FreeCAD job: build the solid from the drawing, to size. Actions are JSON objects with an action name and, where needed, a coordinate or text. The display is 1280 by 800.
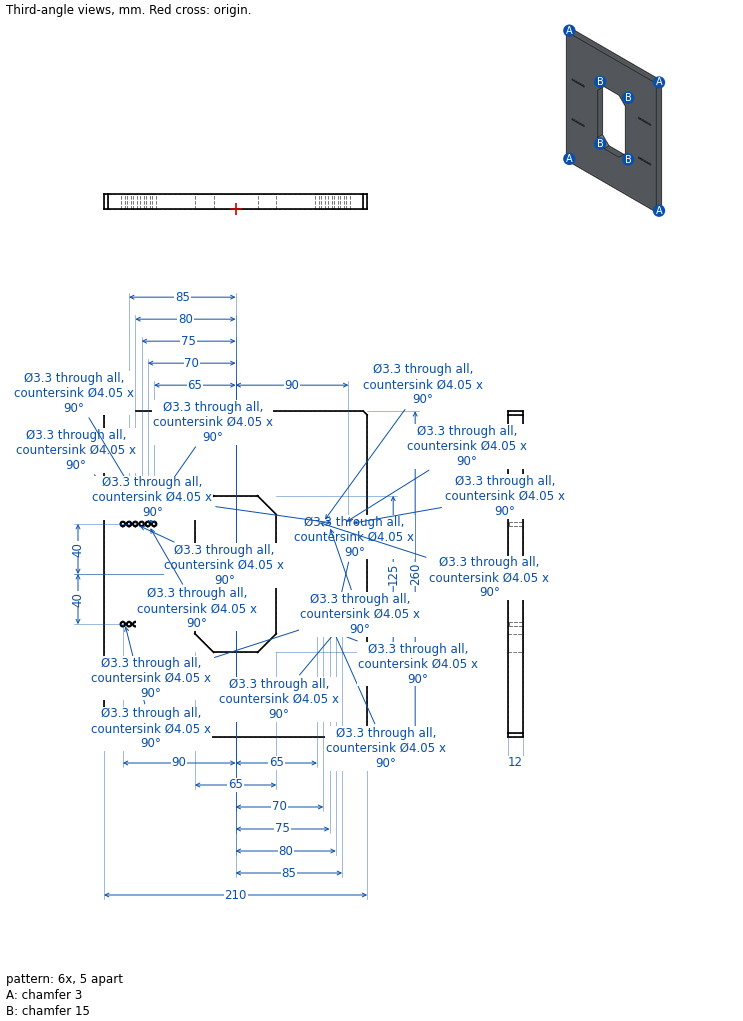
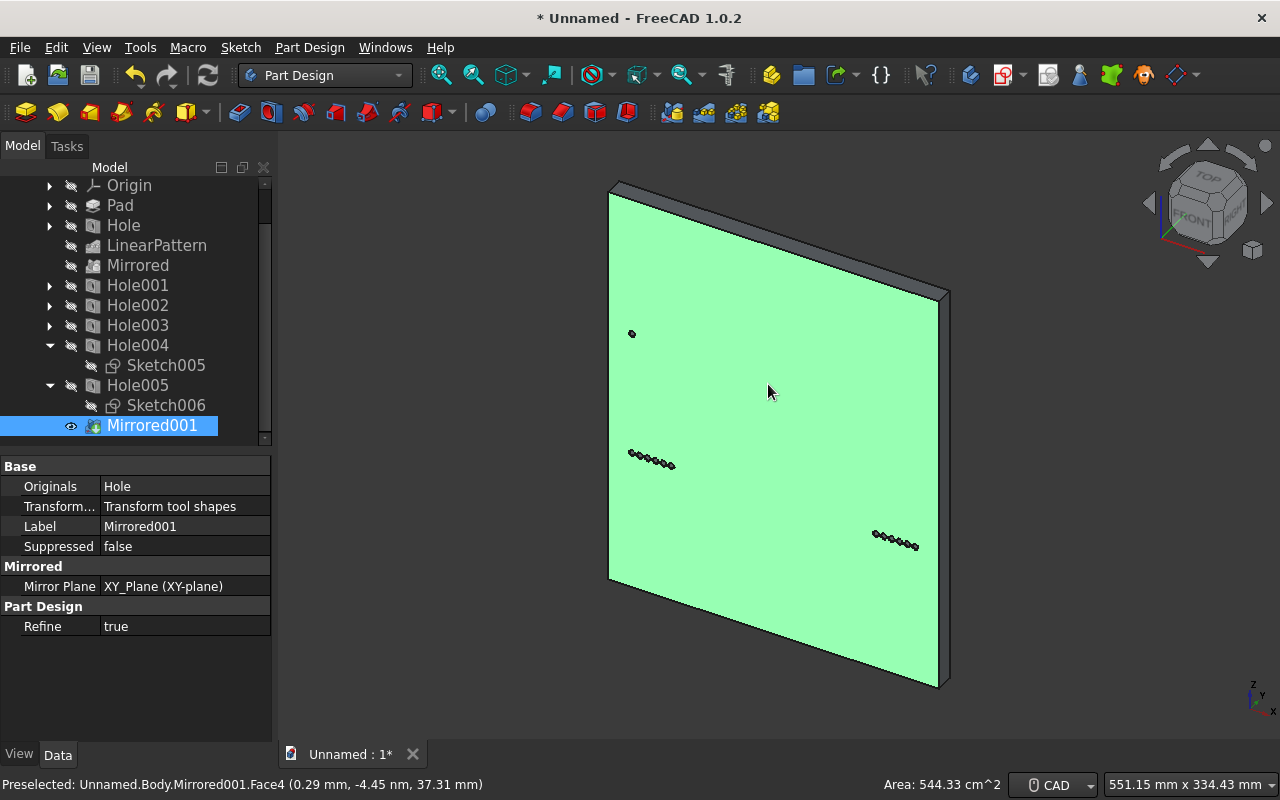
{"action": "left_click", "coordinate": [1004, 76]}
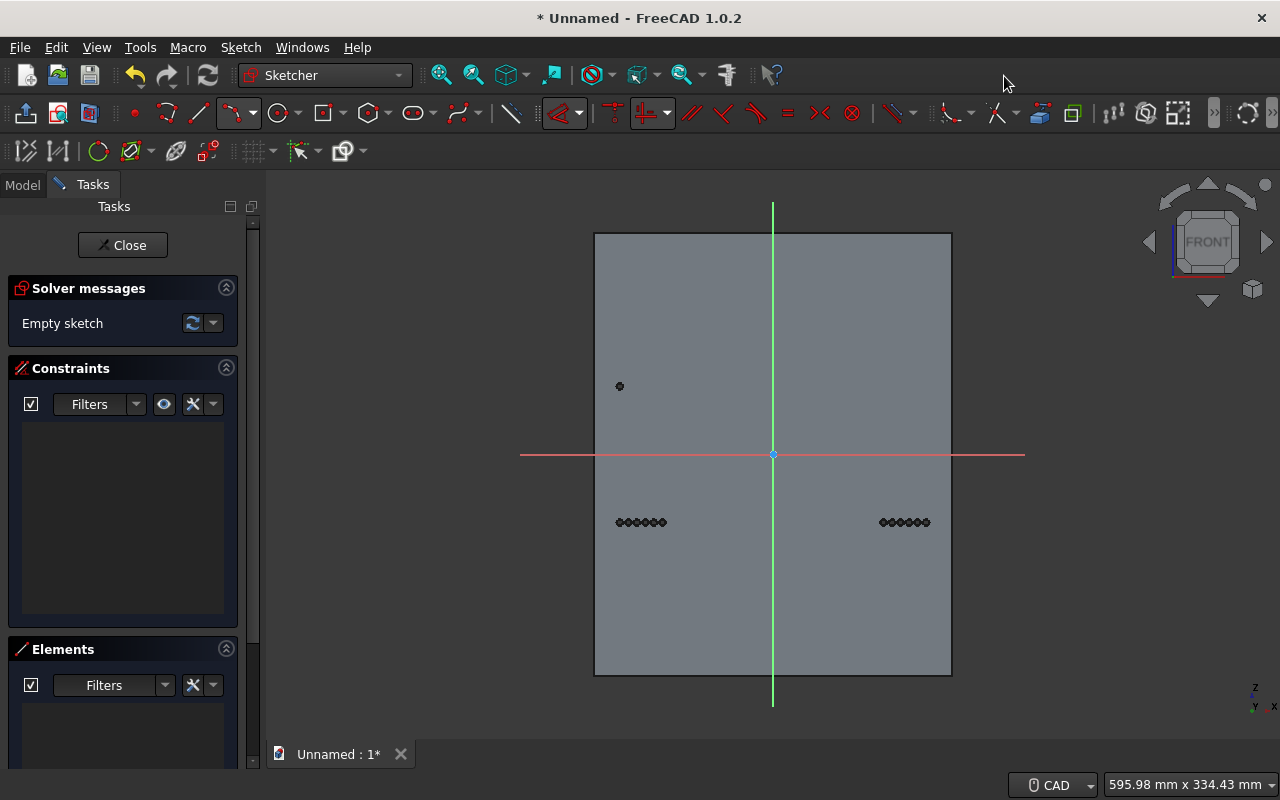
{"action": "scroll", "coordinate": [624, 383], "scroll_direction": "up", "scroll_amount": 15}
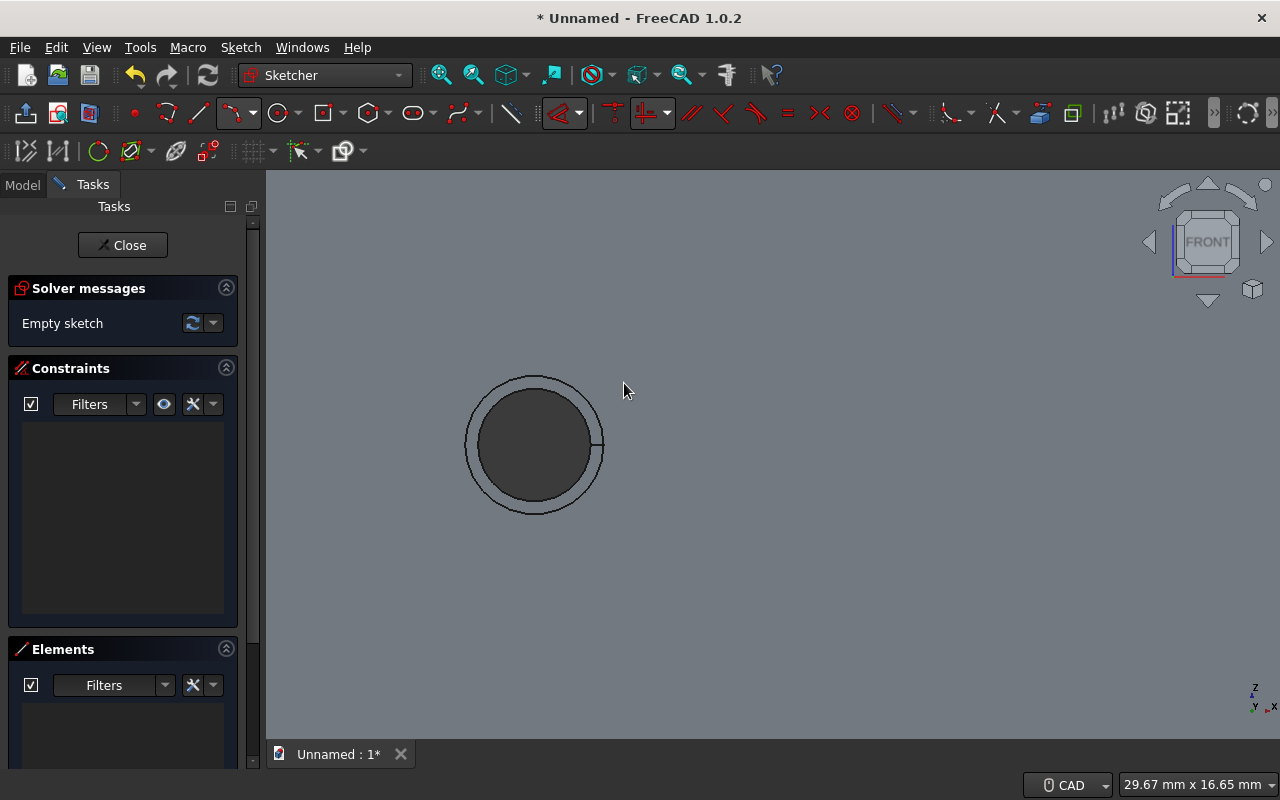
{"action": "scroll", "coordinate": [706, 441], "scroll_direction": "up", "scroll_amount": 6}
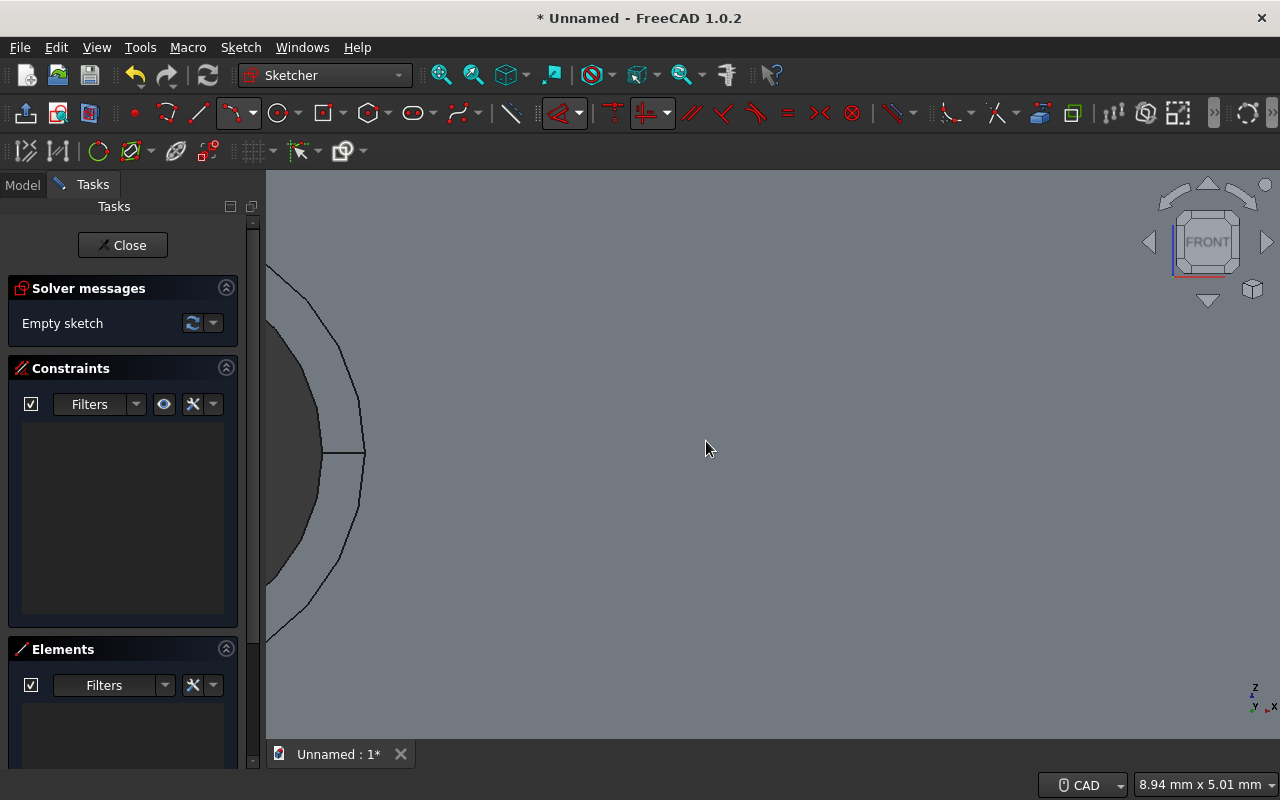
{"action": "left_click", "coordinate": [278, 114]}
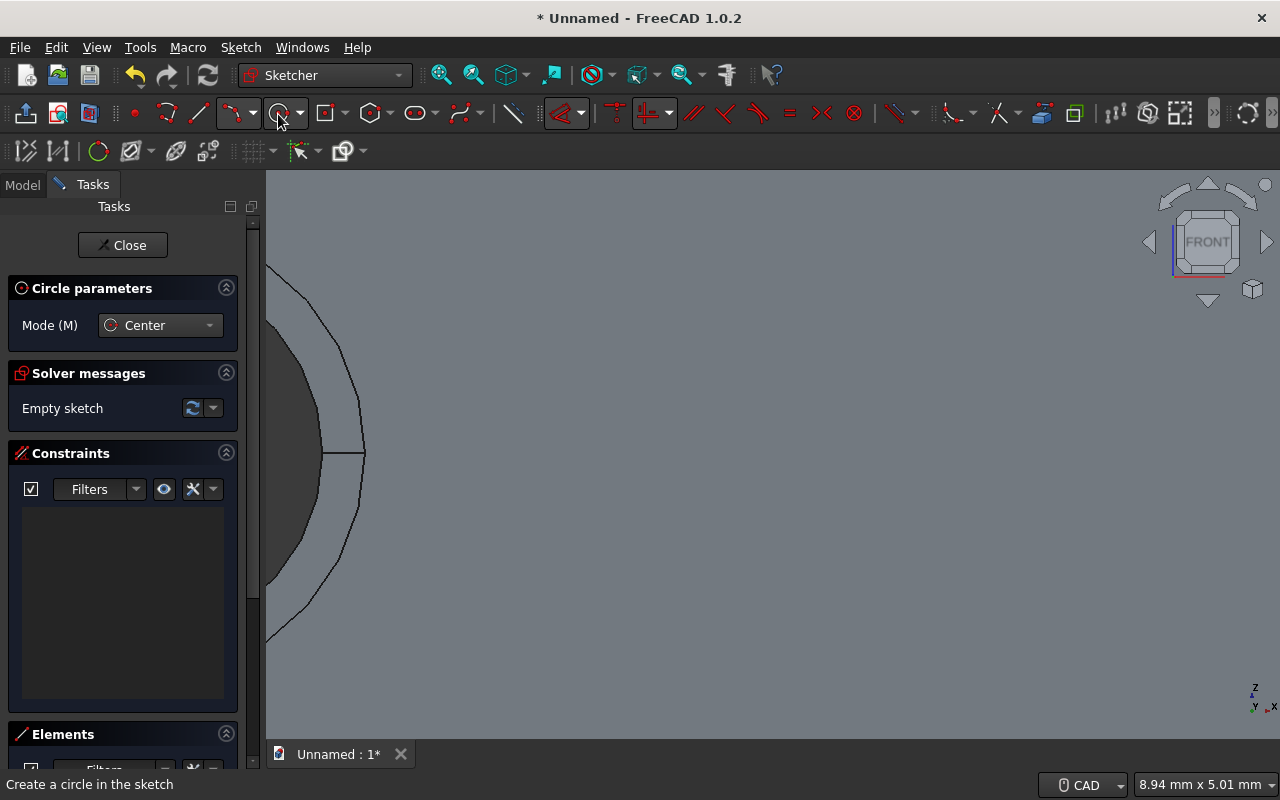
{"action": "left_click", "coordinate": [703, 453]}
{"action": "mouse_move", "coordinate": [835, 321]}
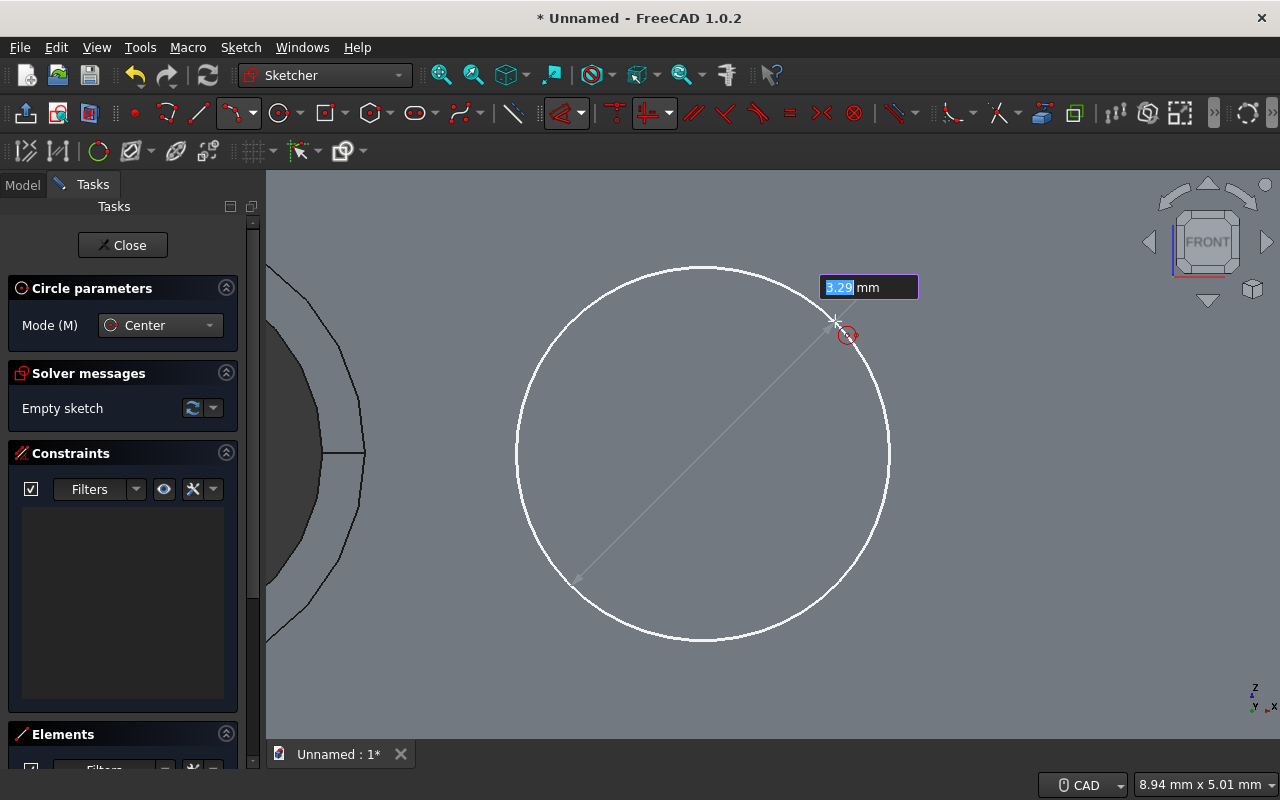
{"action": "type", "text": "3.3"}
{"action": "key", "text": "Return"}
{"action": "key", "text": "Escape"}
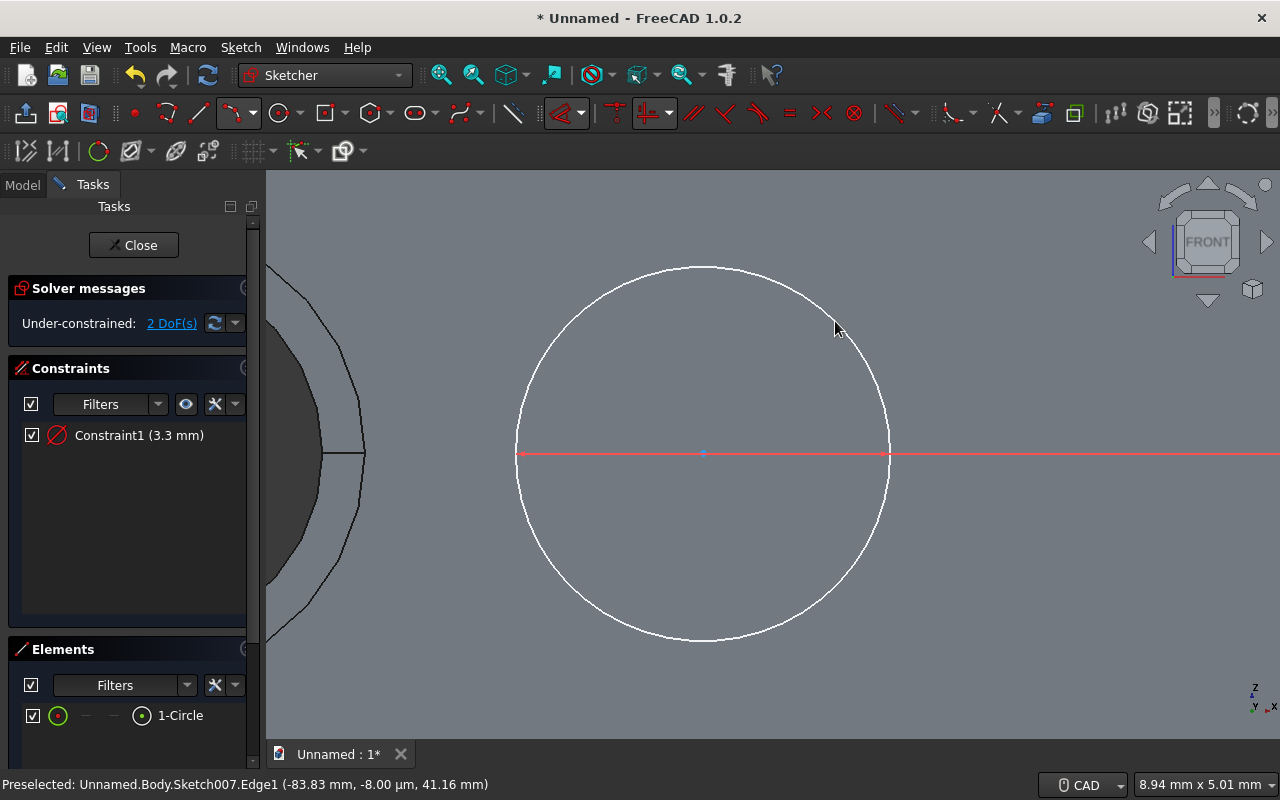
{"action": "left_click", "coordinate": [703, 454]}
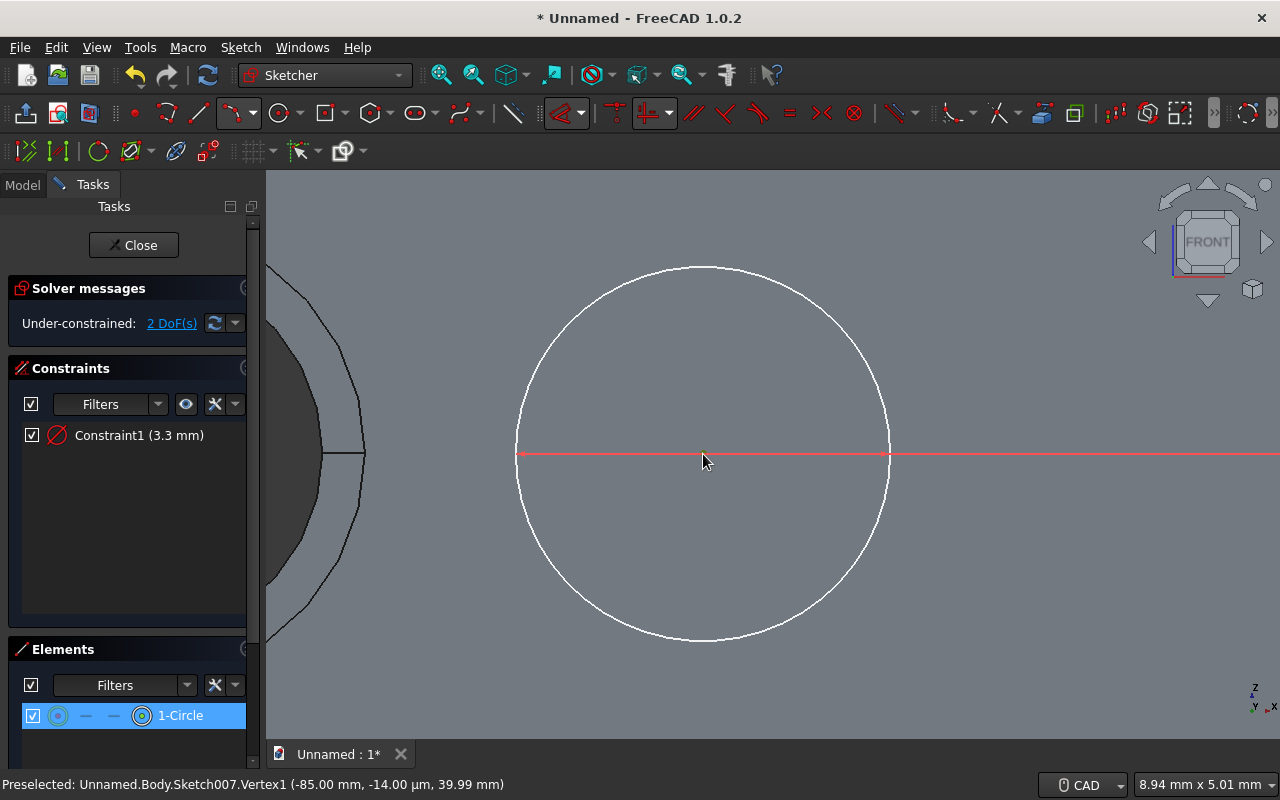
{"action": "left_click", "coordinate": [584, 114]}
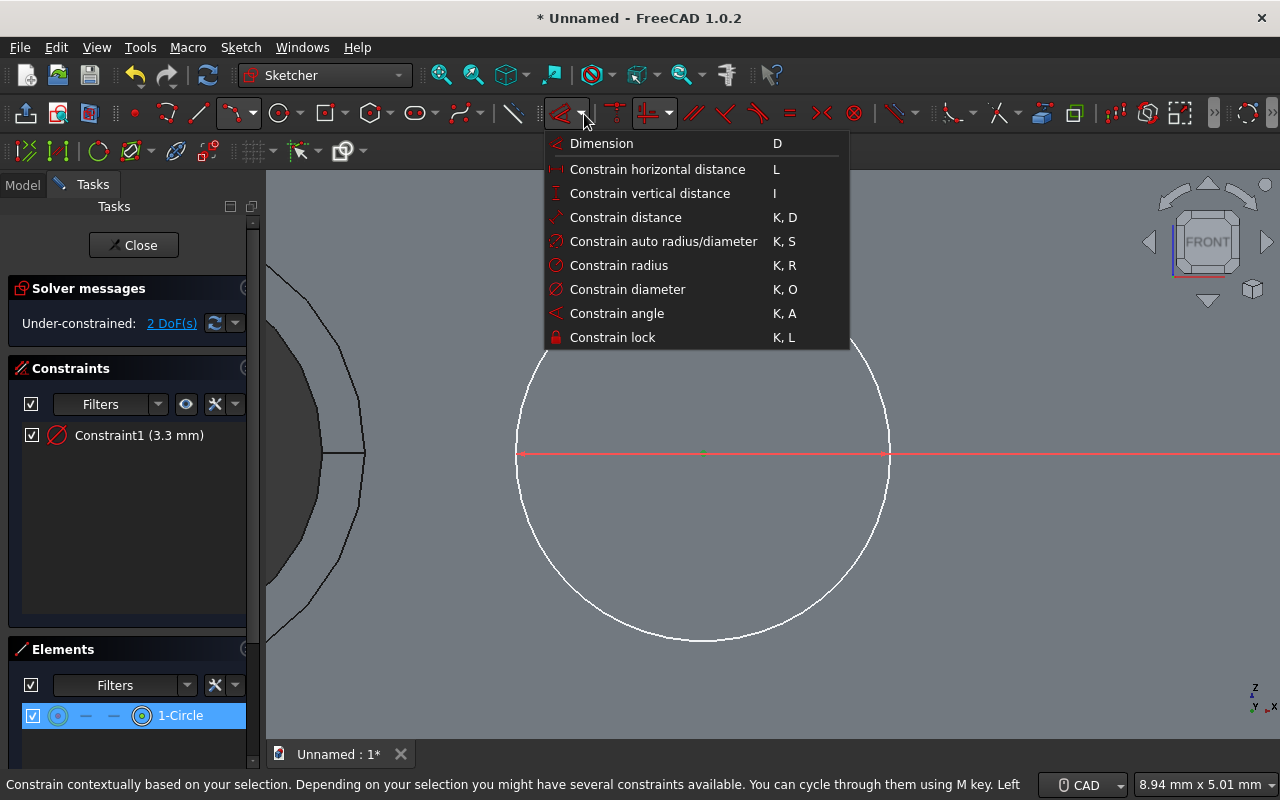
{"action": "left_click", "coordinate": [697, 169]}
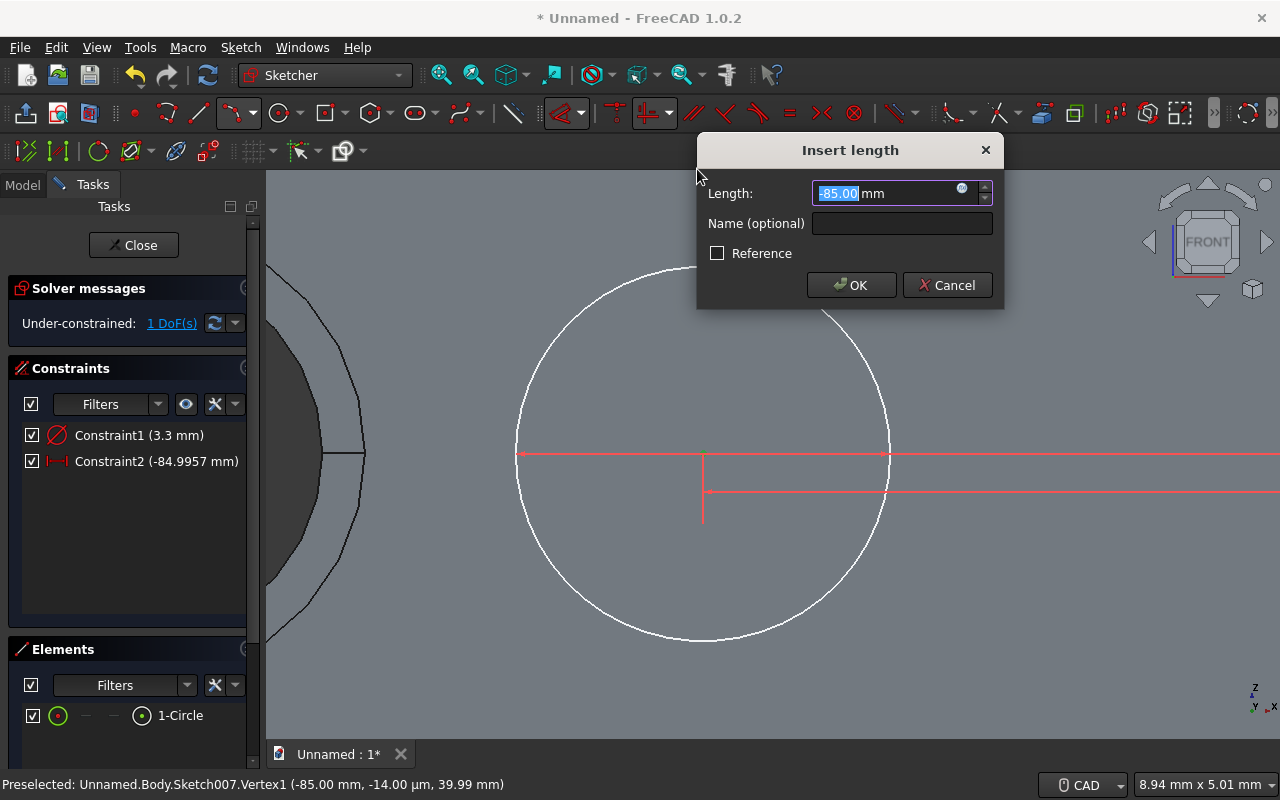
{"action": "type", "text": "-85"}
{"action": "key", "text": "Return"}